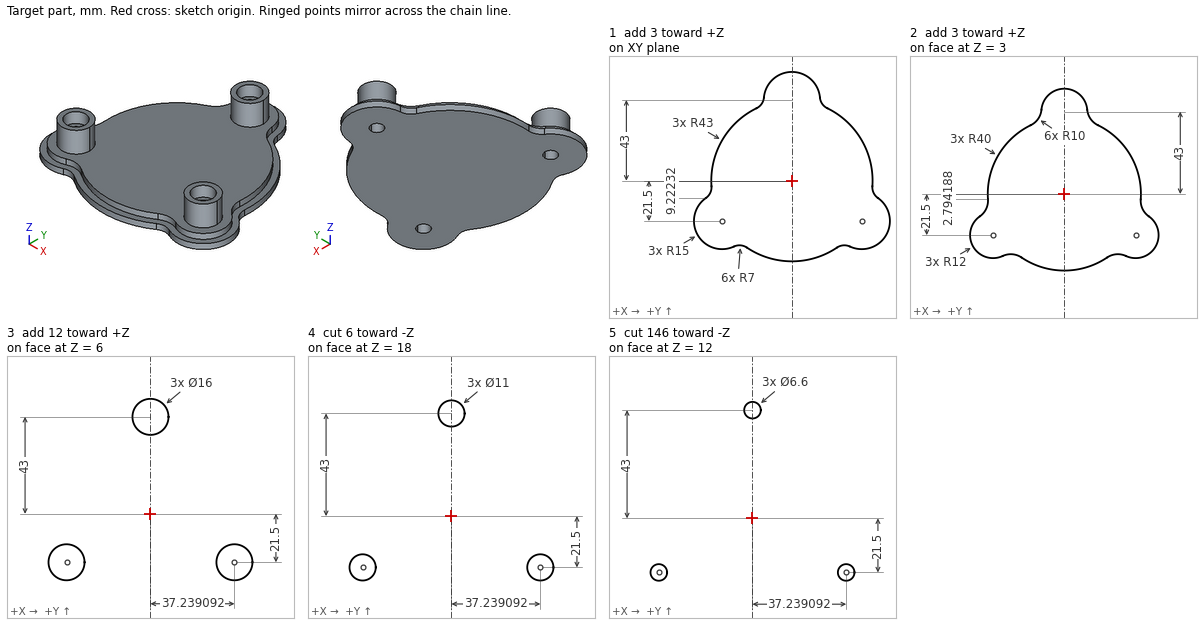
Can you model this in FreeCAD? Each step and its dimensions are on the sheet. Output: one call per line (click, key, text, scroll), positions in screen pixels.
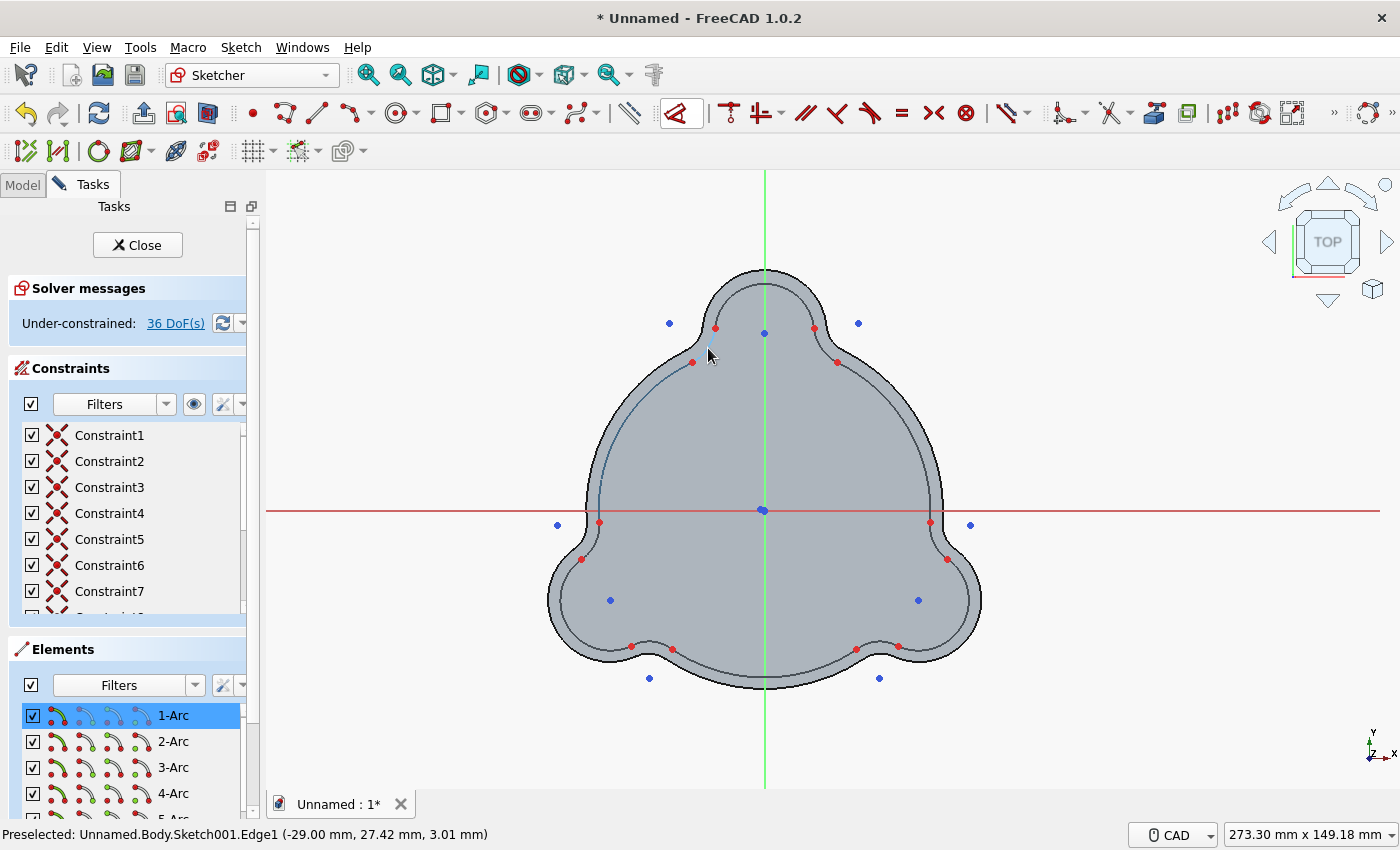
click(591, 551)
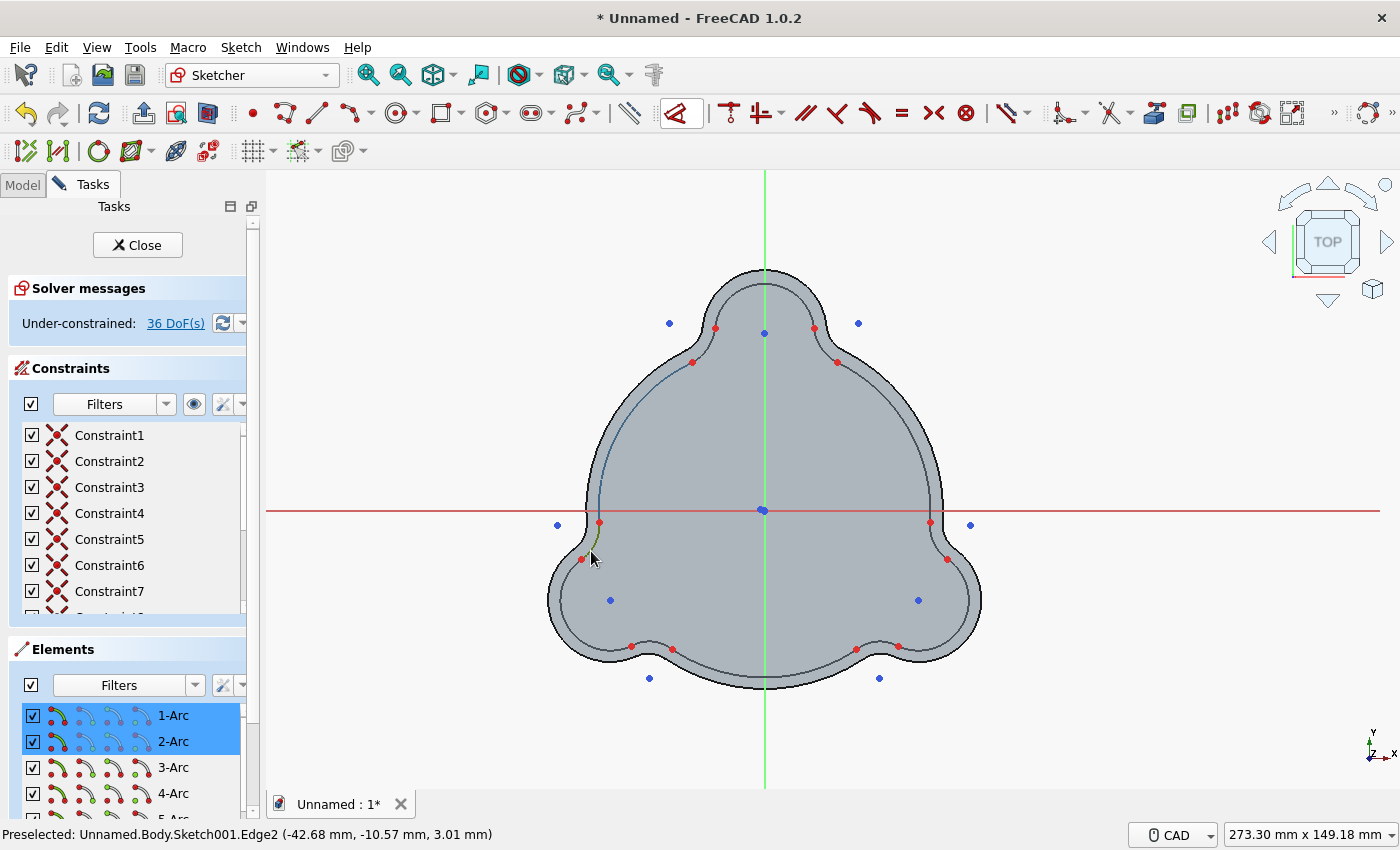
click(870, 114)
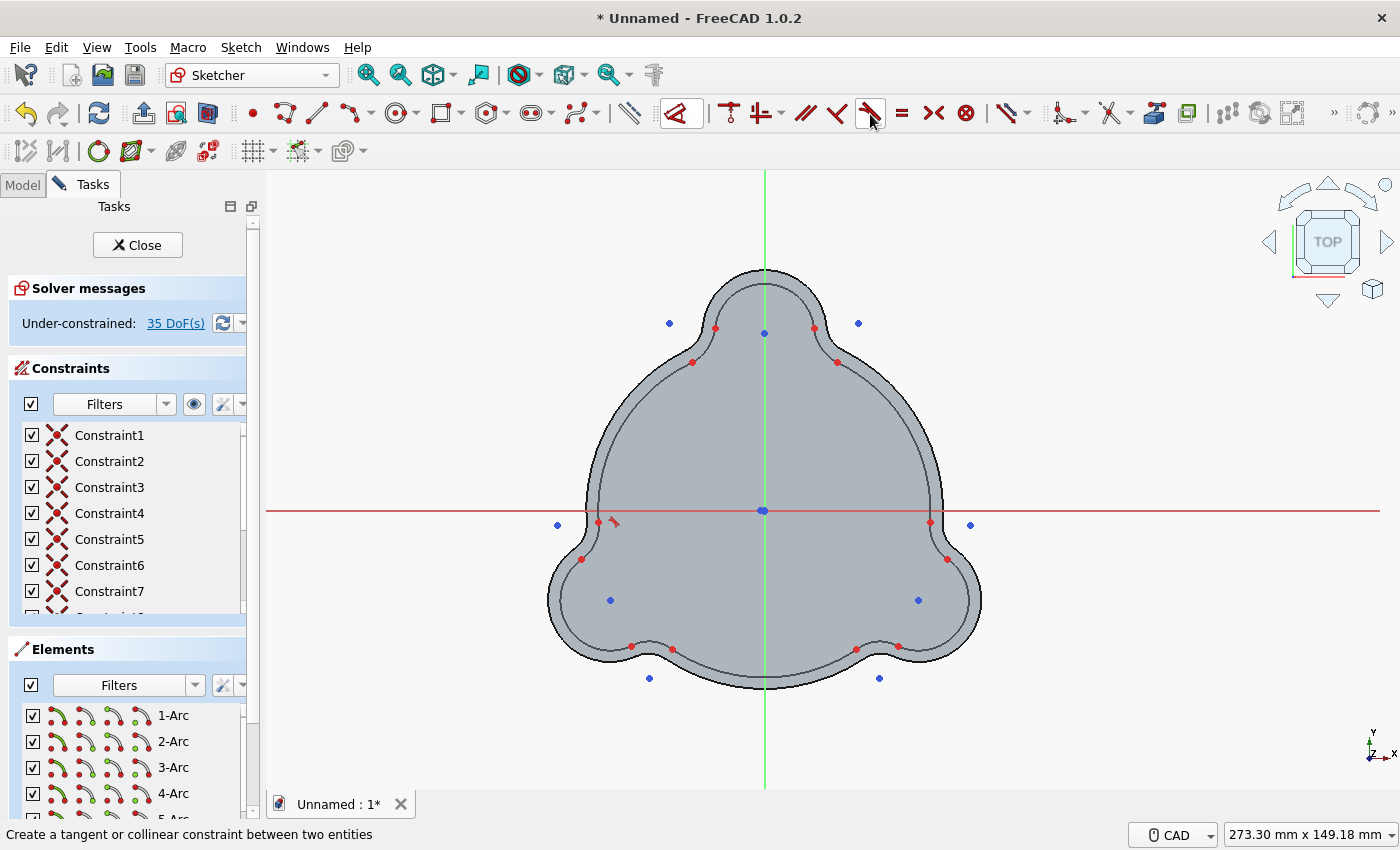
click(644, 397)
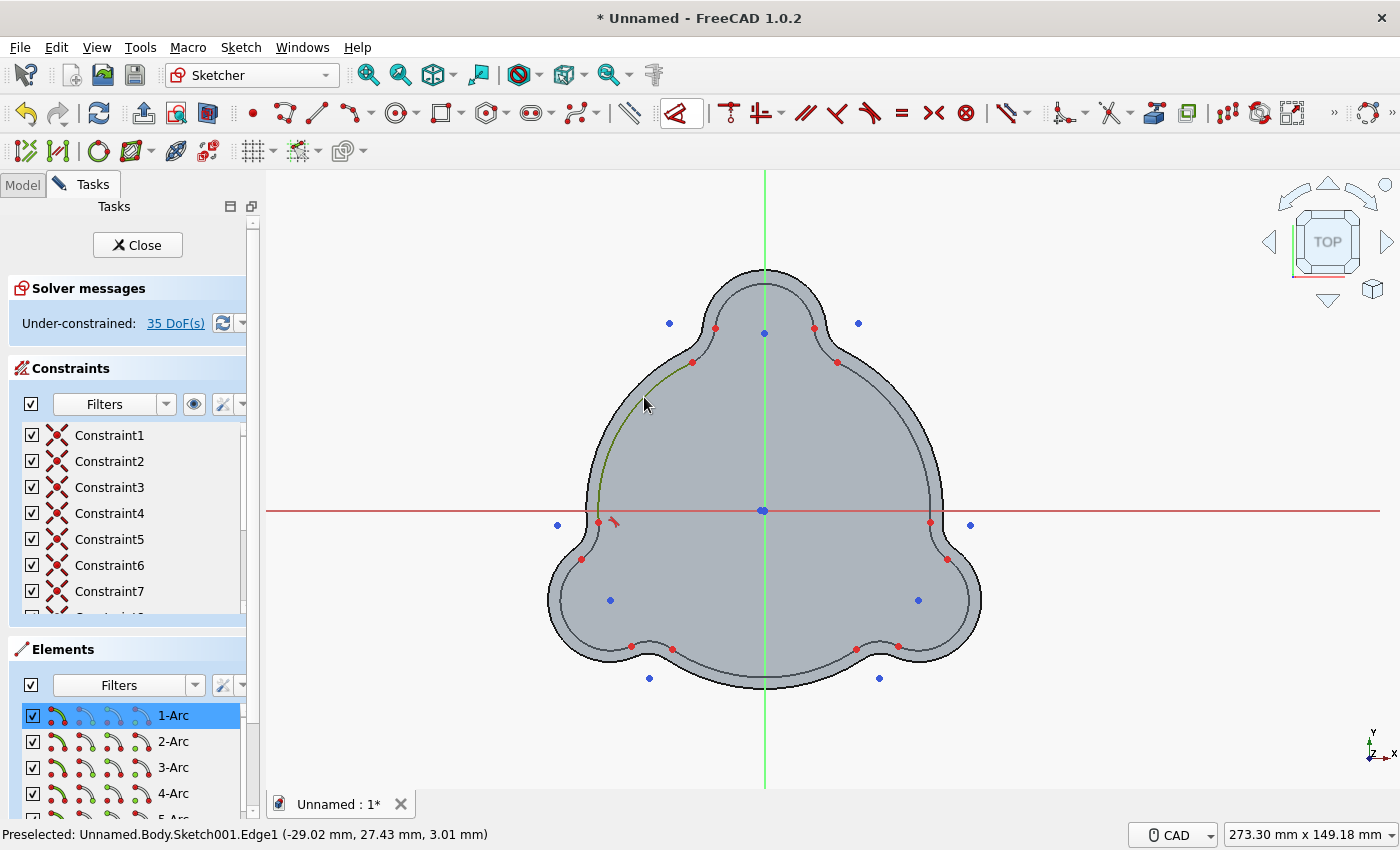
click(702, 355)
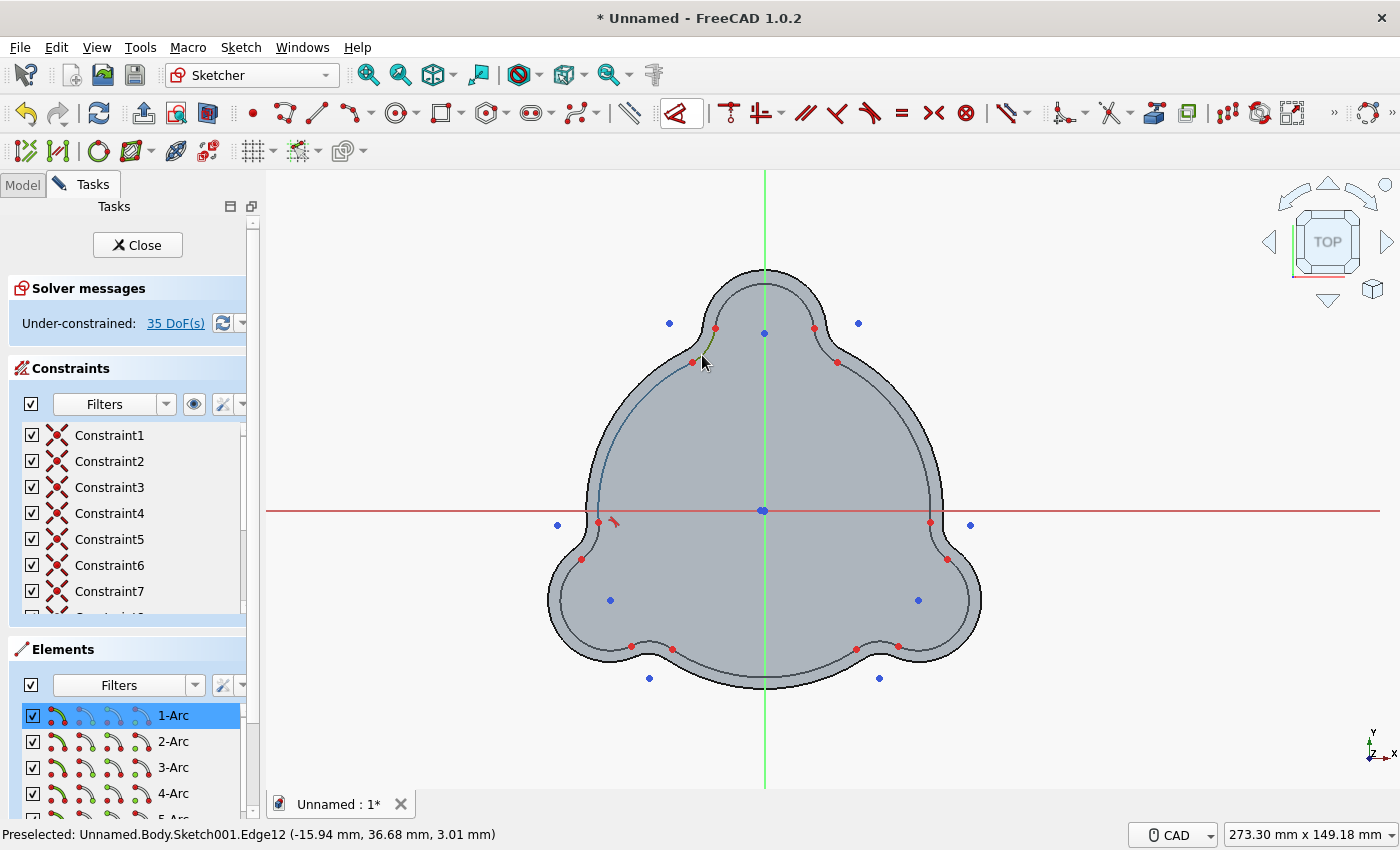
key(t)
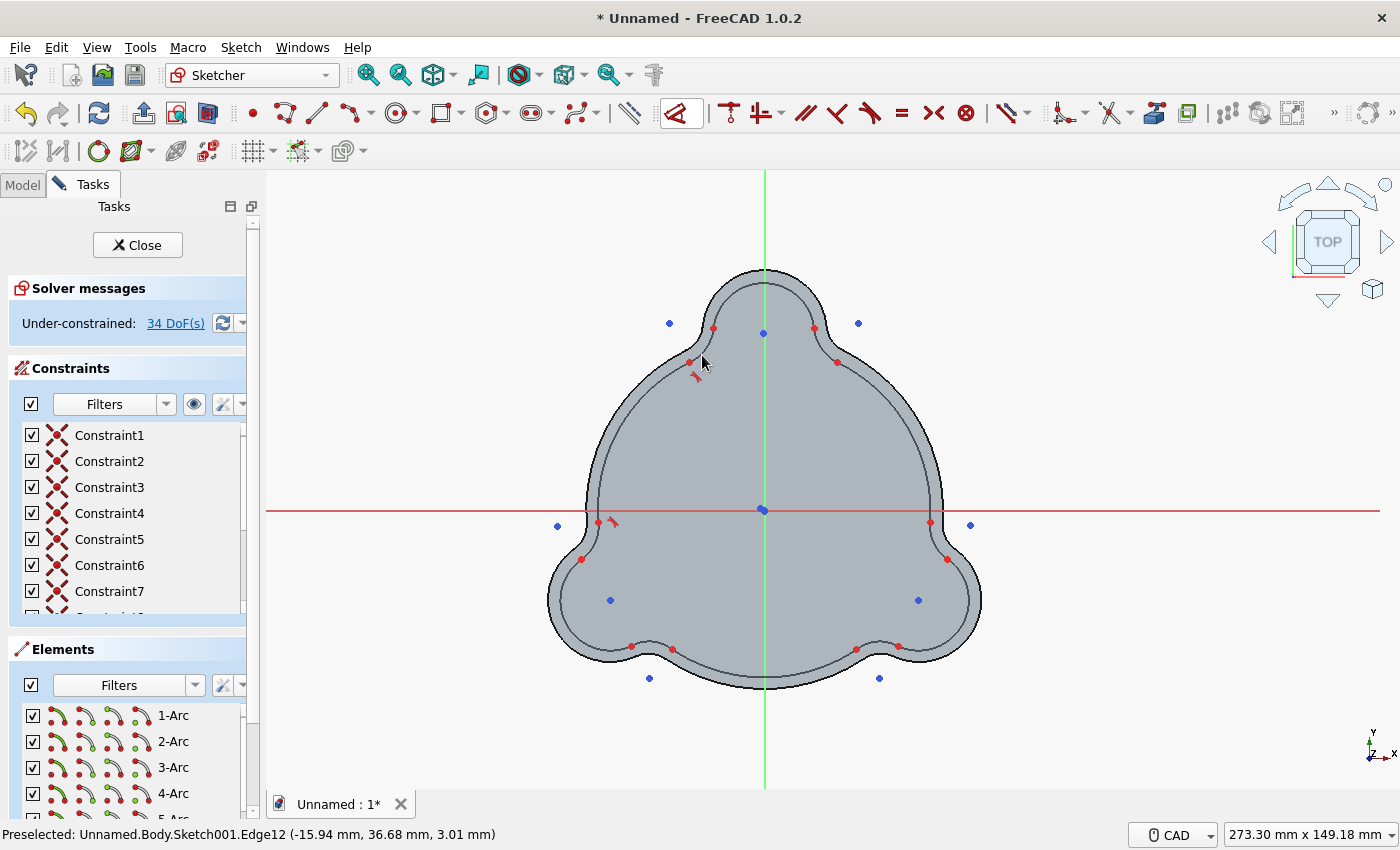
click(591, 551)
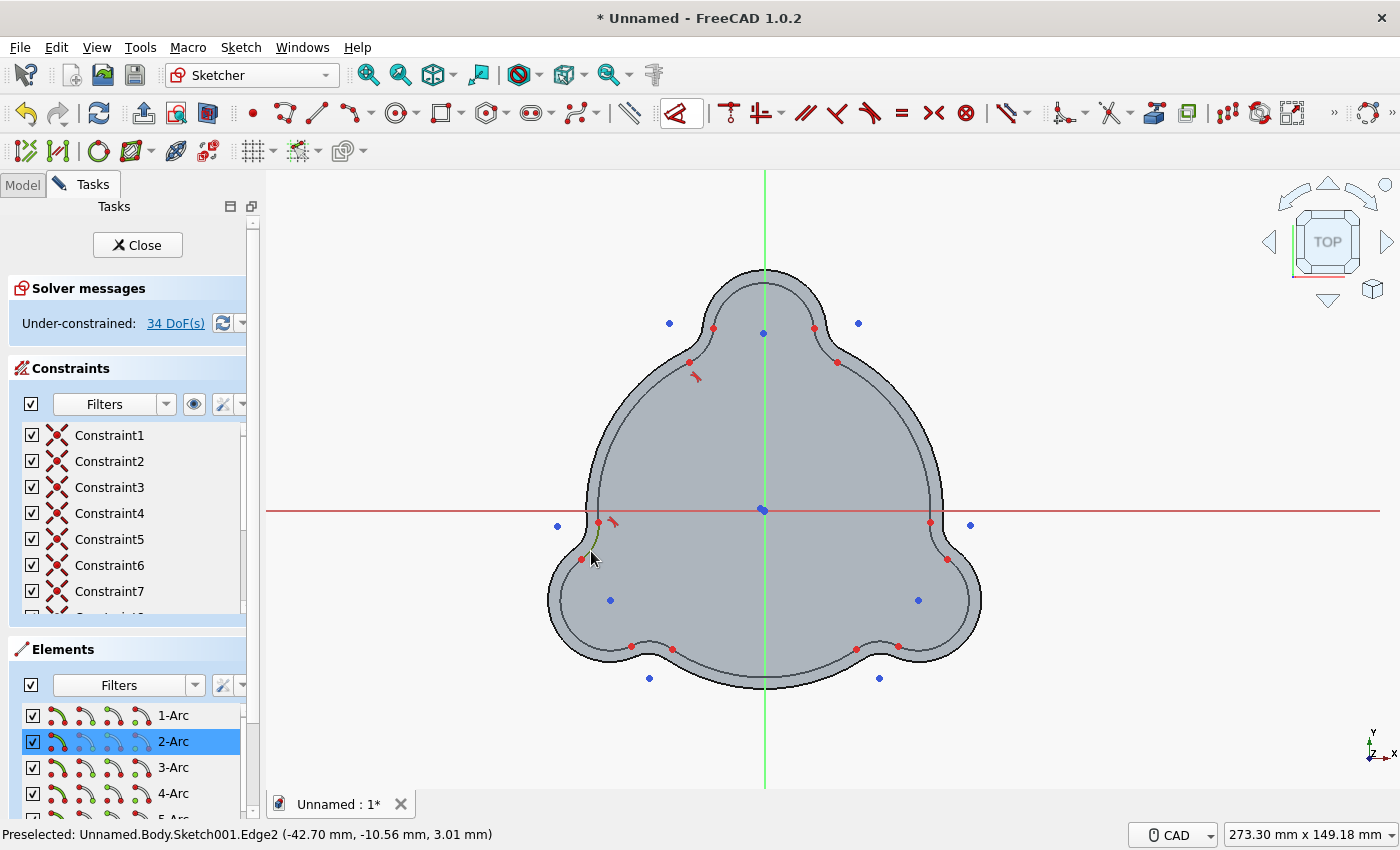
click(561, 597)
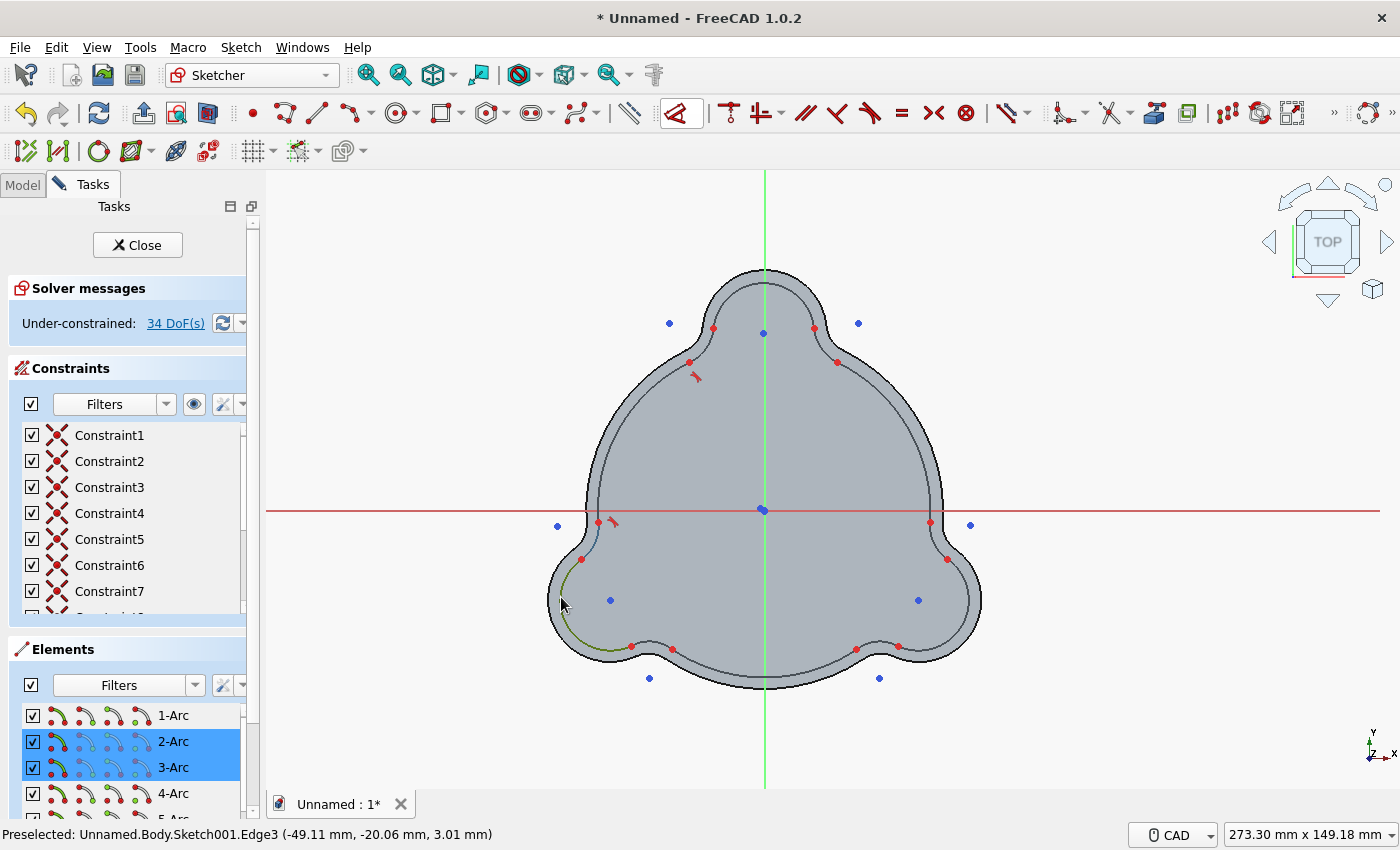
click(870, 114)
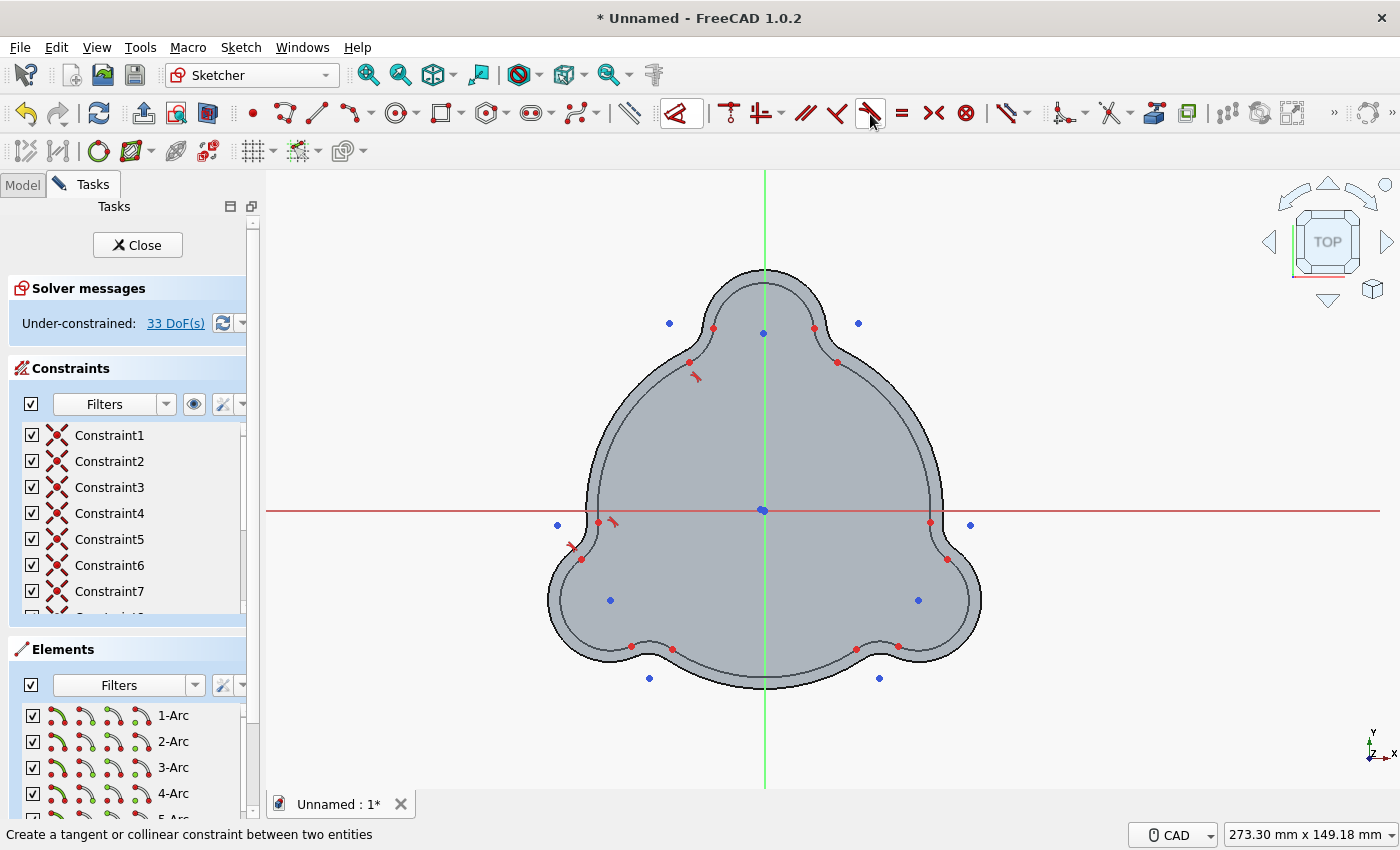
click(560, 597)